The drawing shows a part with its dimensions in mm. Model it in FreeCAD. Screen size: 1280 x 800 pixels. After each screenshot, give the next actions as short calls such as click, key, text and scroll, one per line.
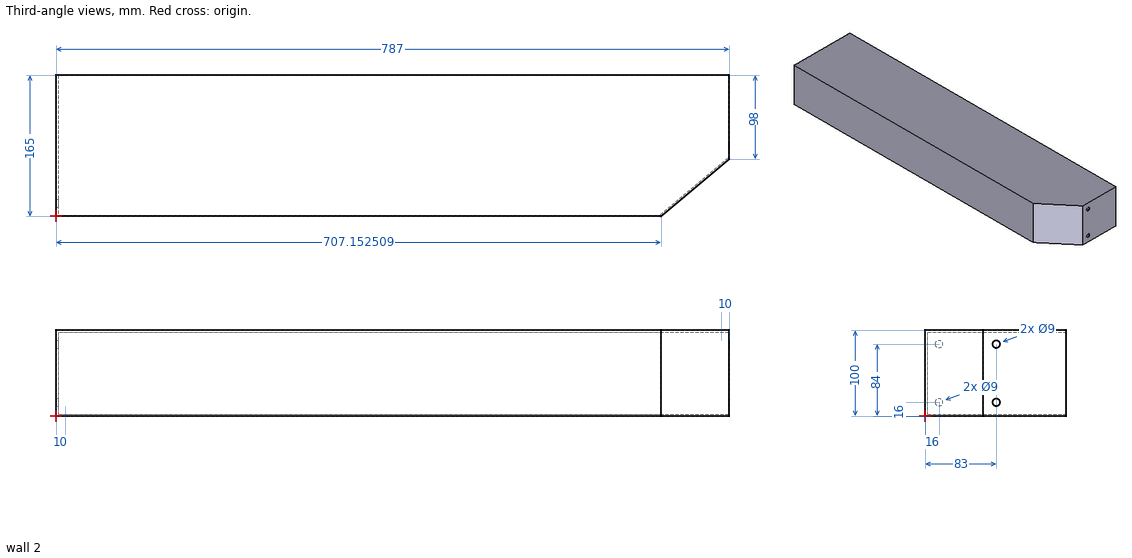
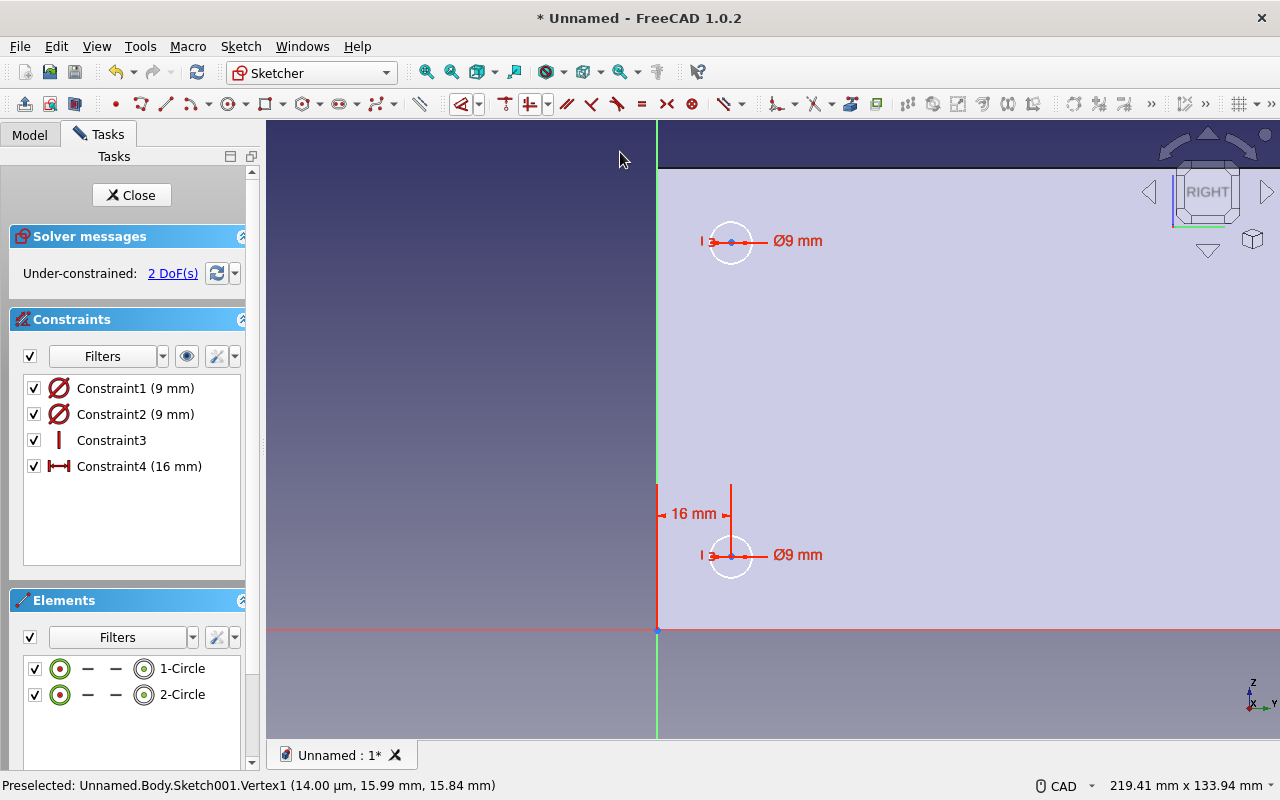
click(731, 557)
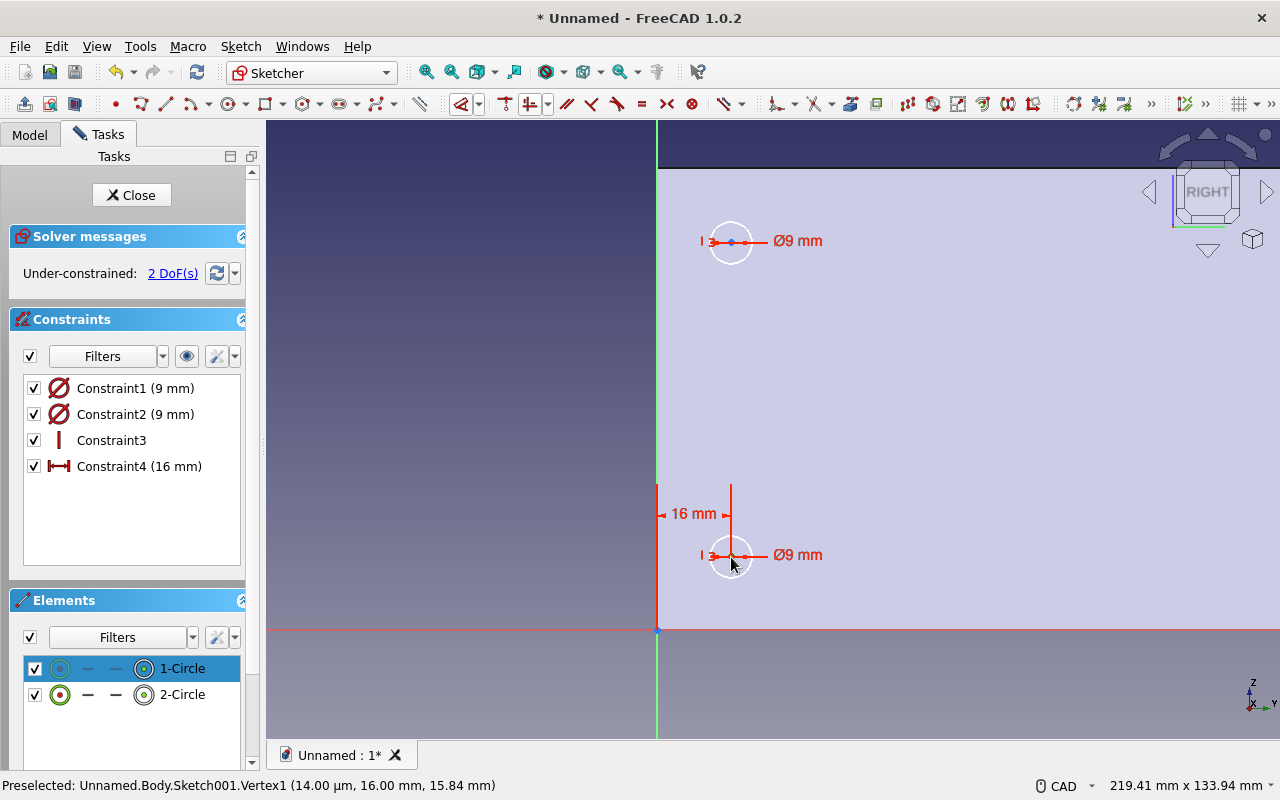
click(478, 104)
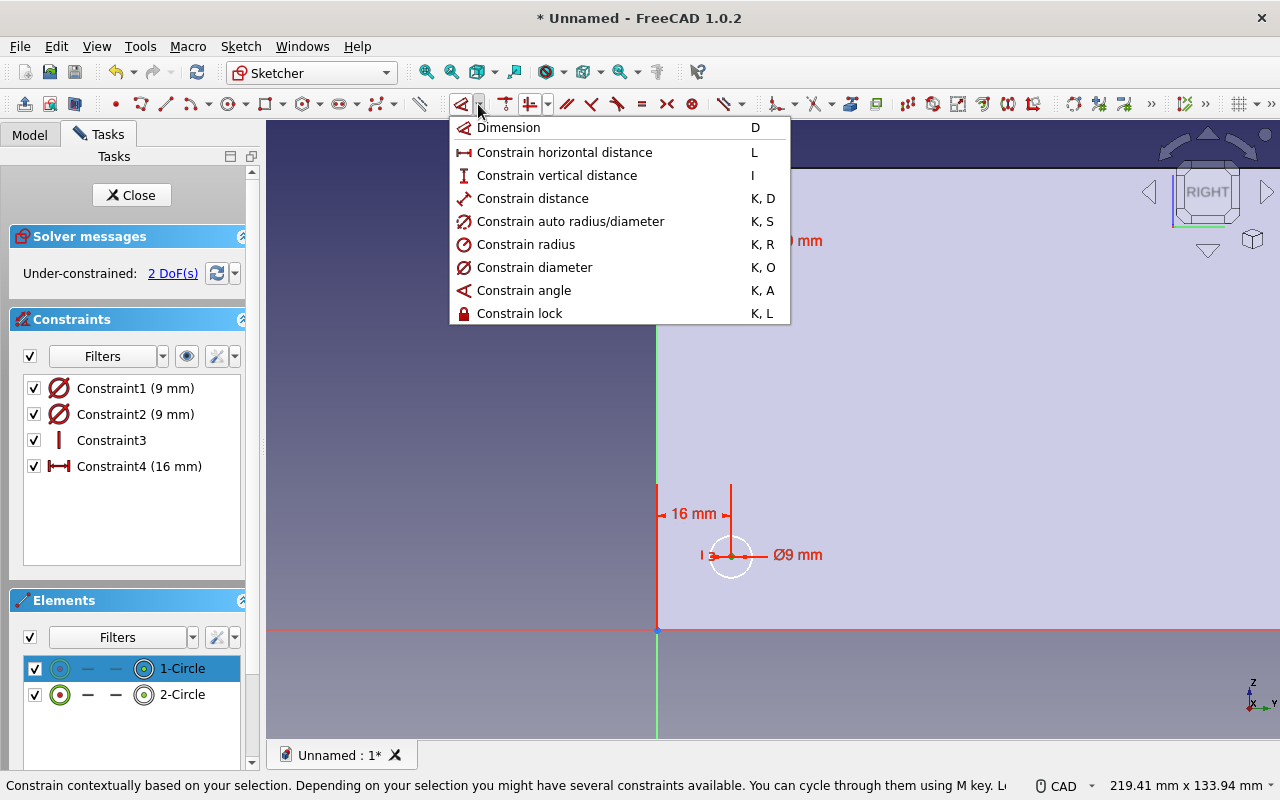
click(620, 176)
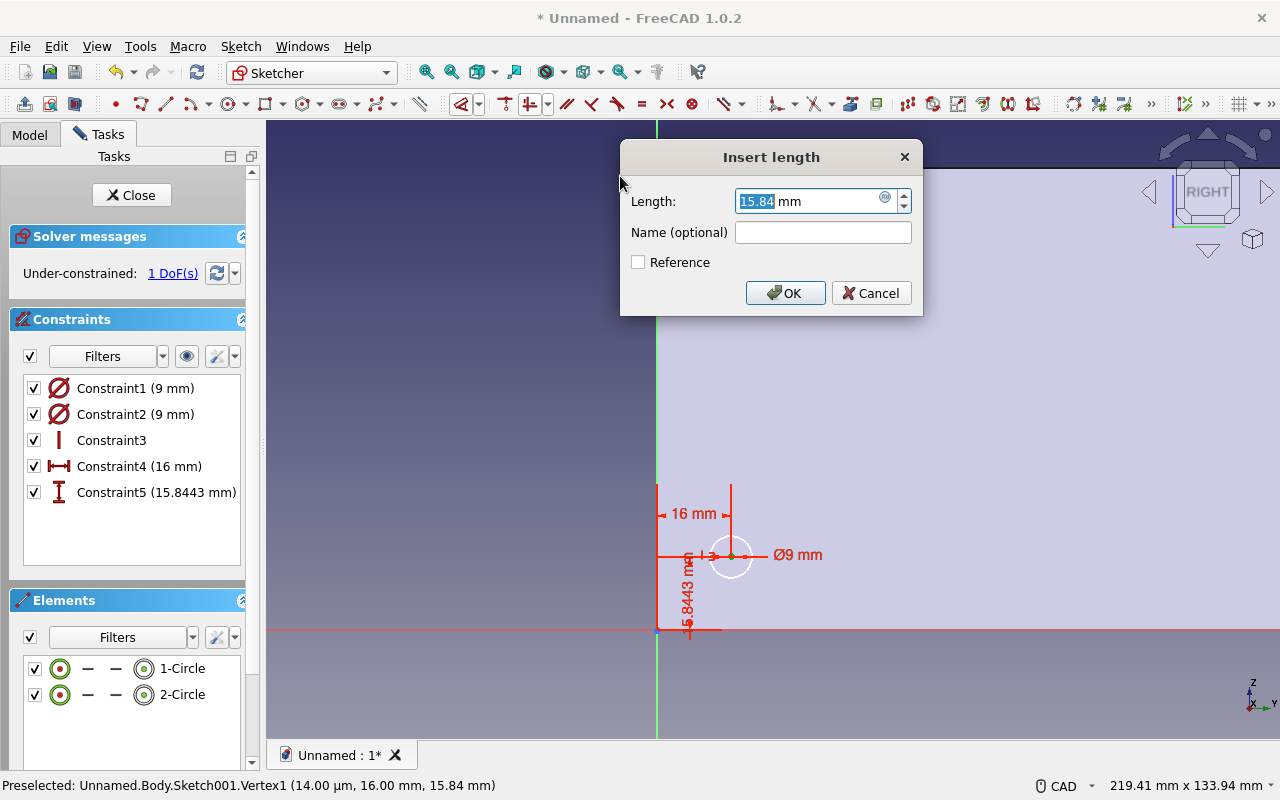
text(16)
key(Return)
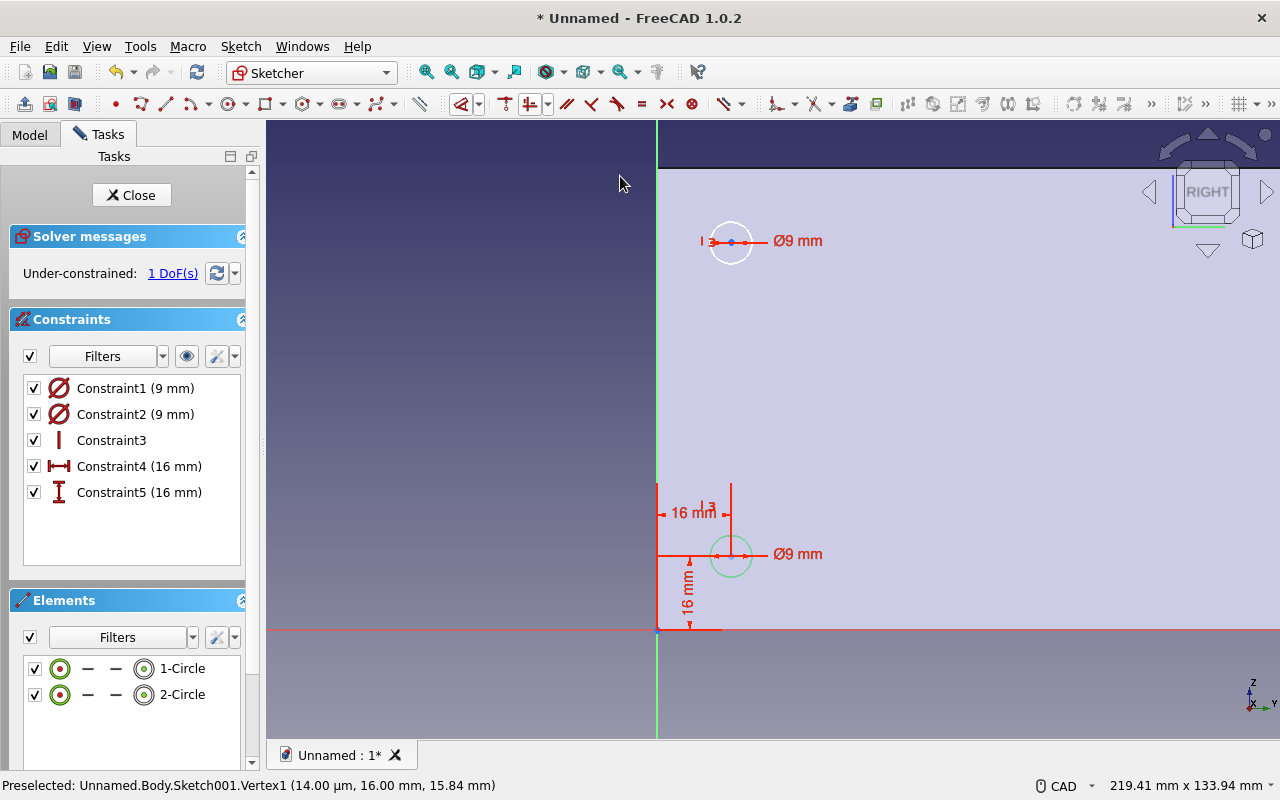
click(731, 243)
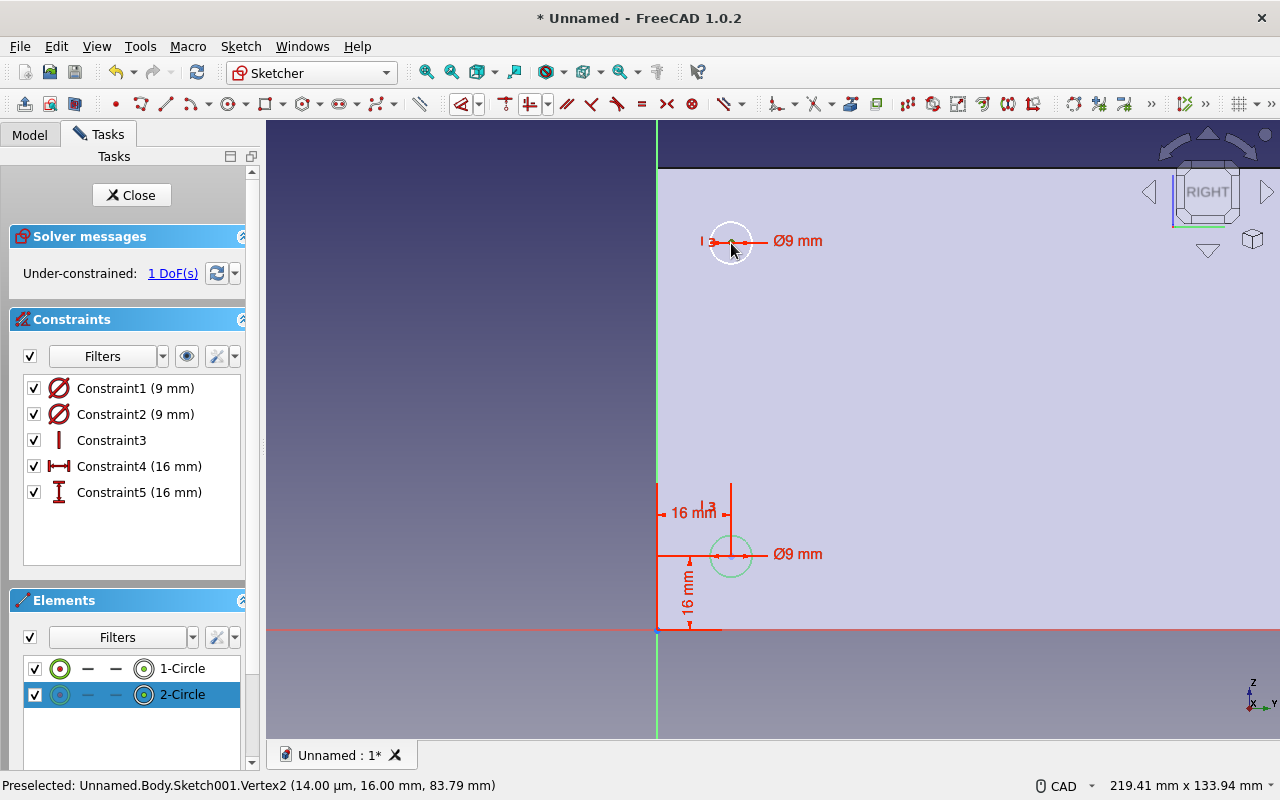
click(478, 104)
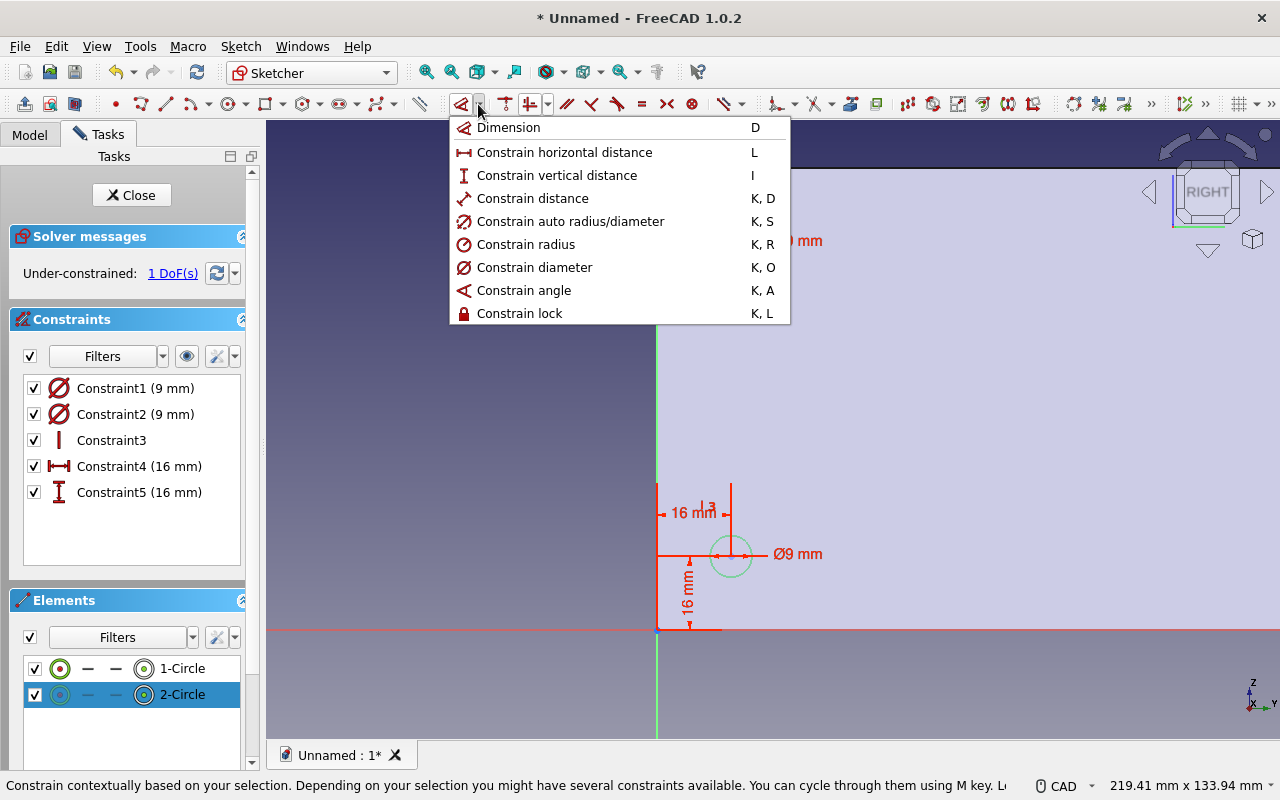
click(620, 176)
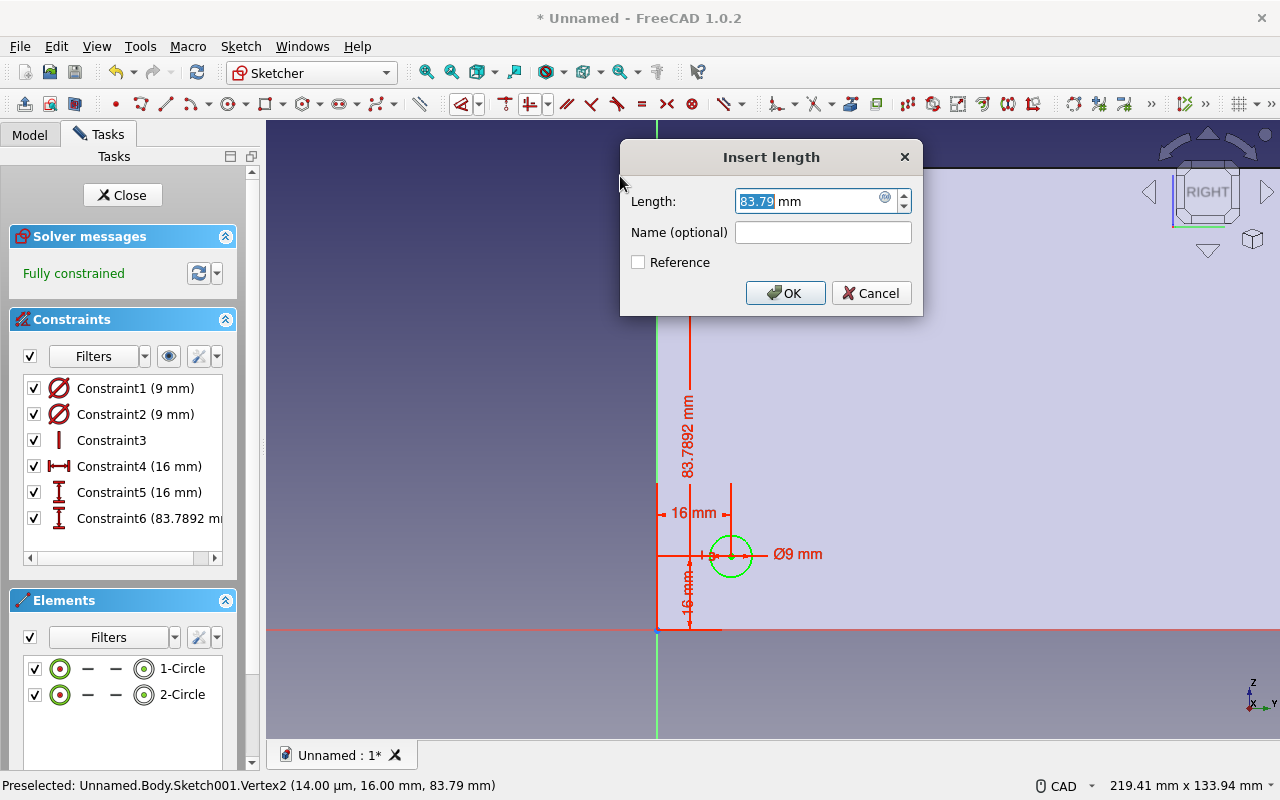
text(84)
key(Return)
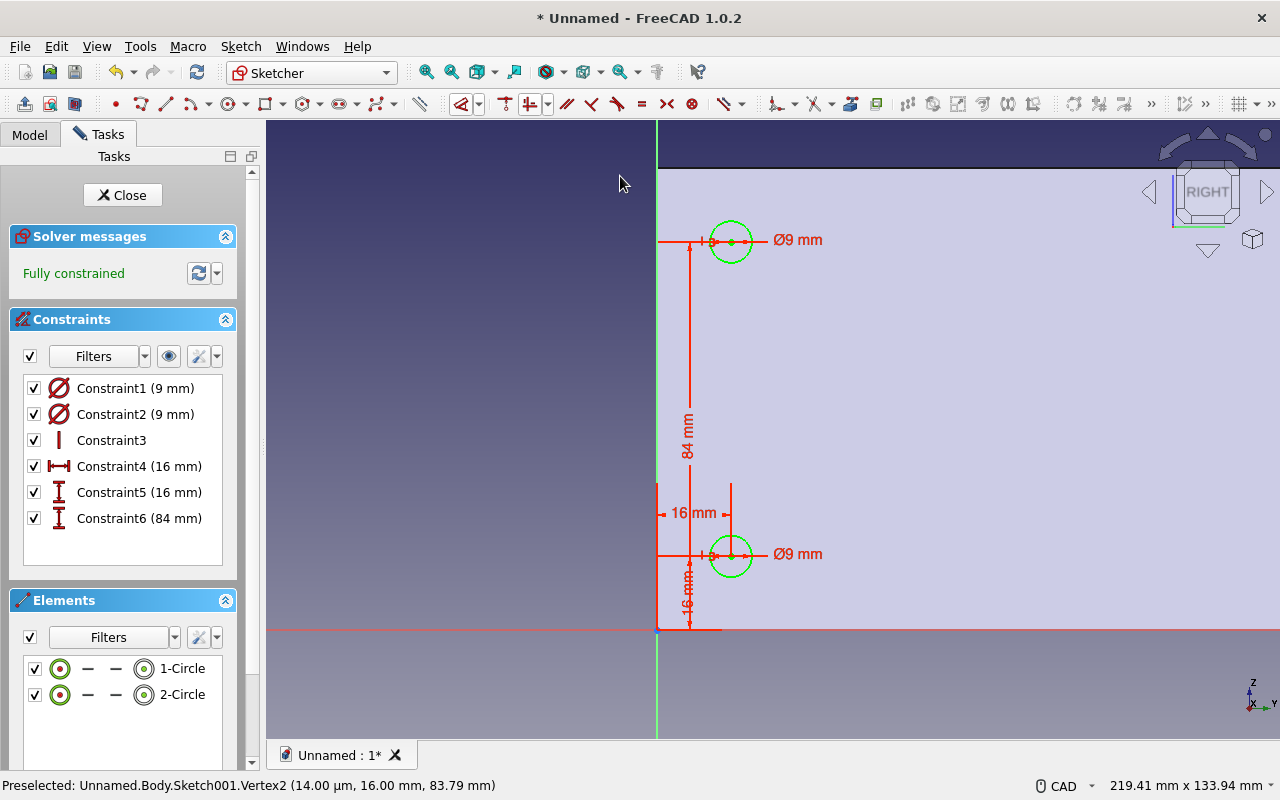
click(123, 195)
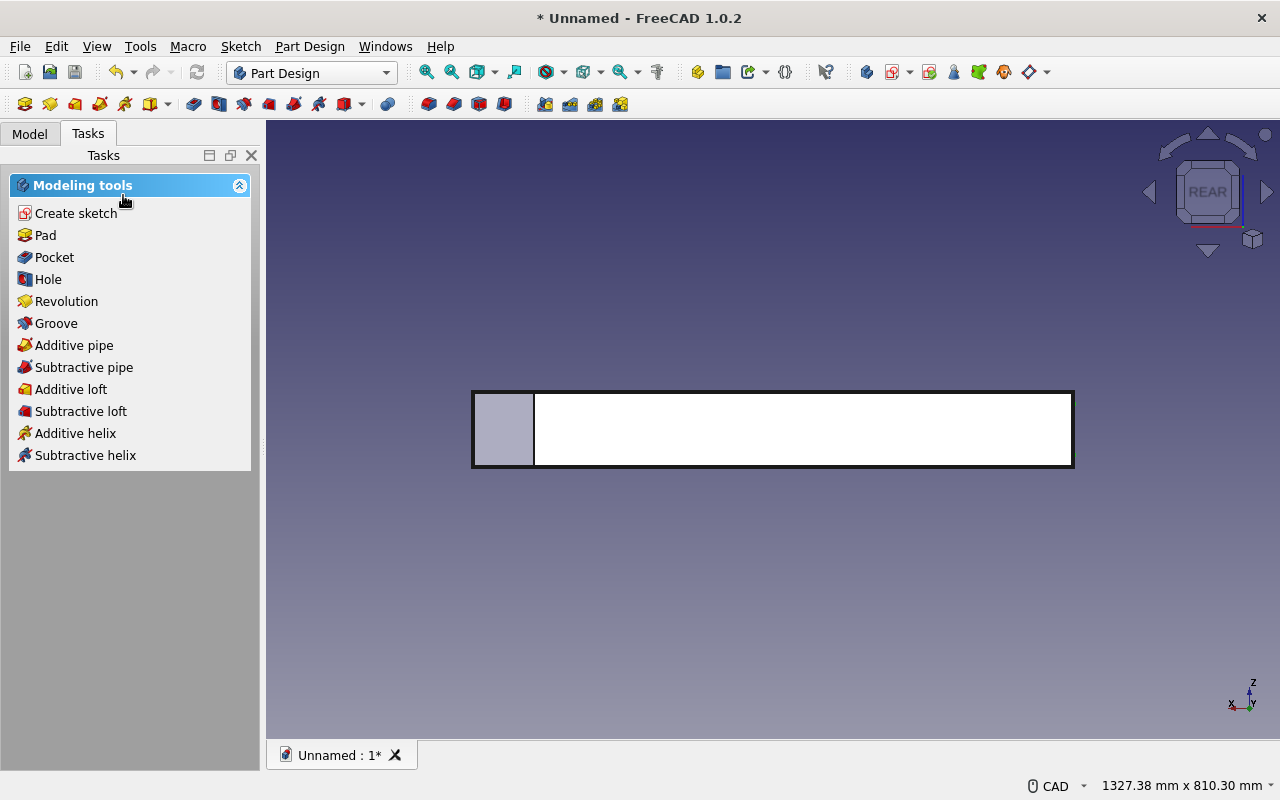
click(194, 104)